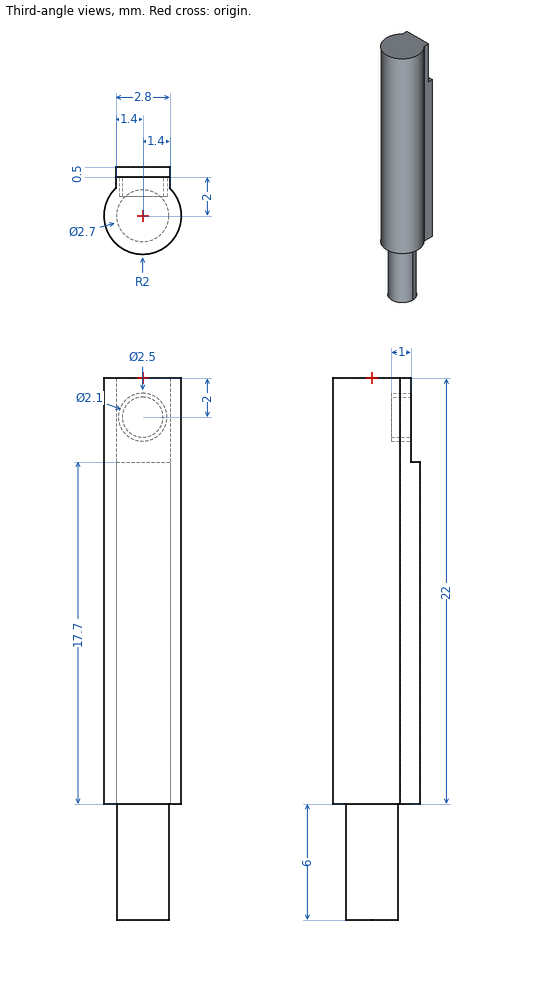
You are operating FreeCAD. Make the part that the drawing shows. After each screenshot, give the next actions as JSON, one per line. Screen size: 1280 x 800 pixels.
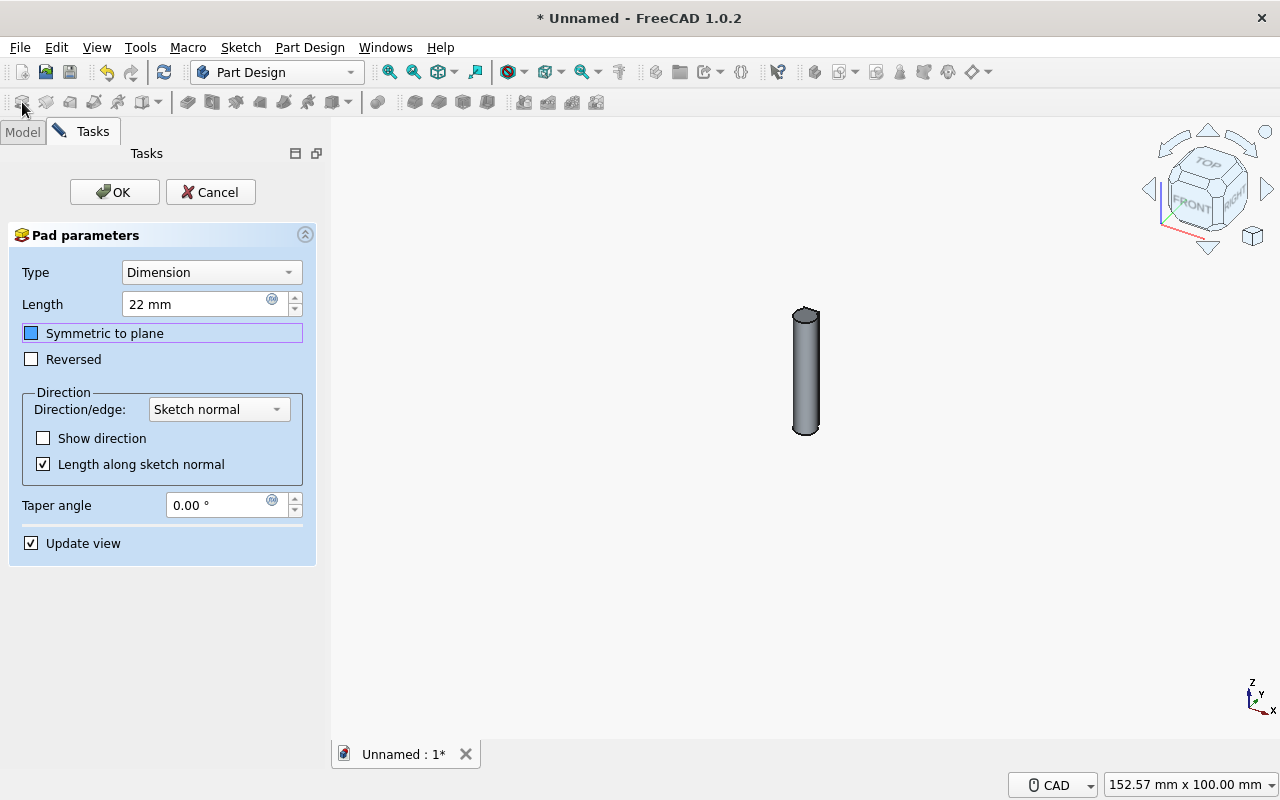
{"action": "left_click", "coordinate": [30, 359]}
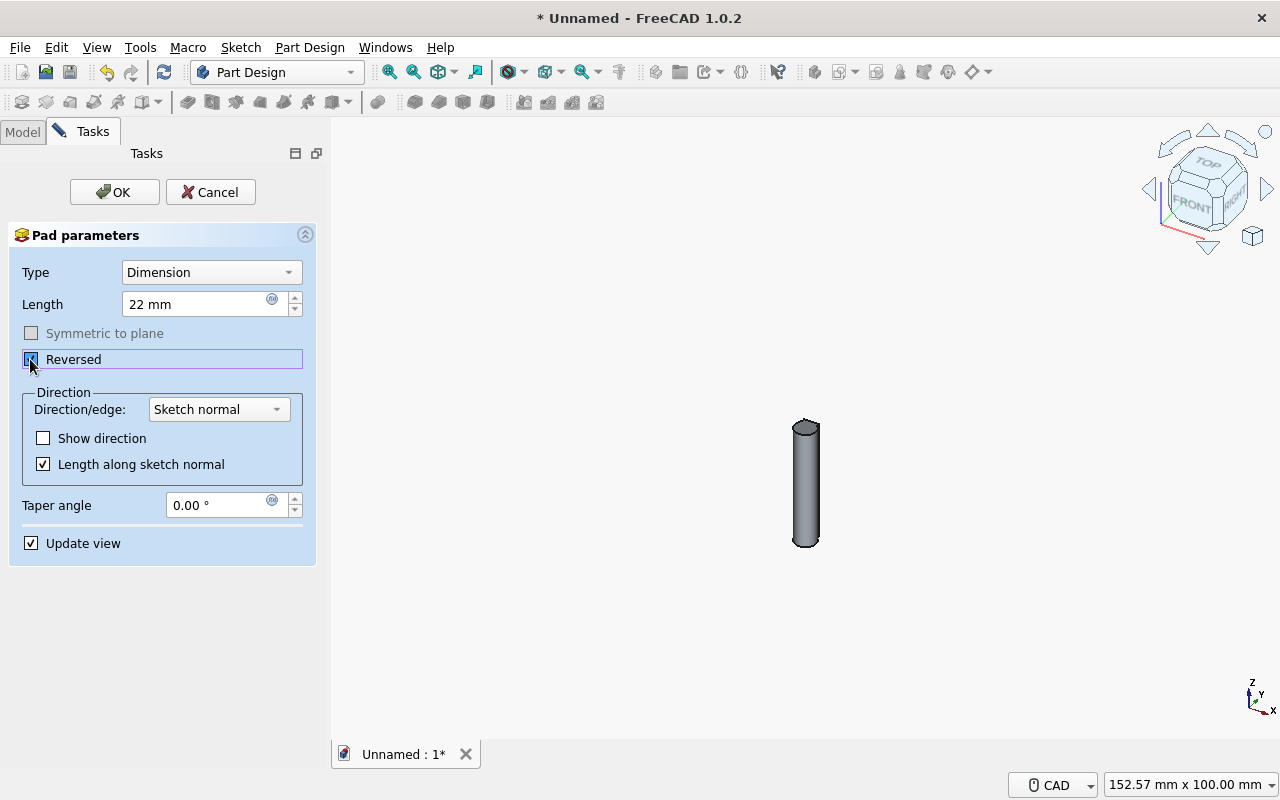
{"action": "left_click", "coordinate": [115, 192]}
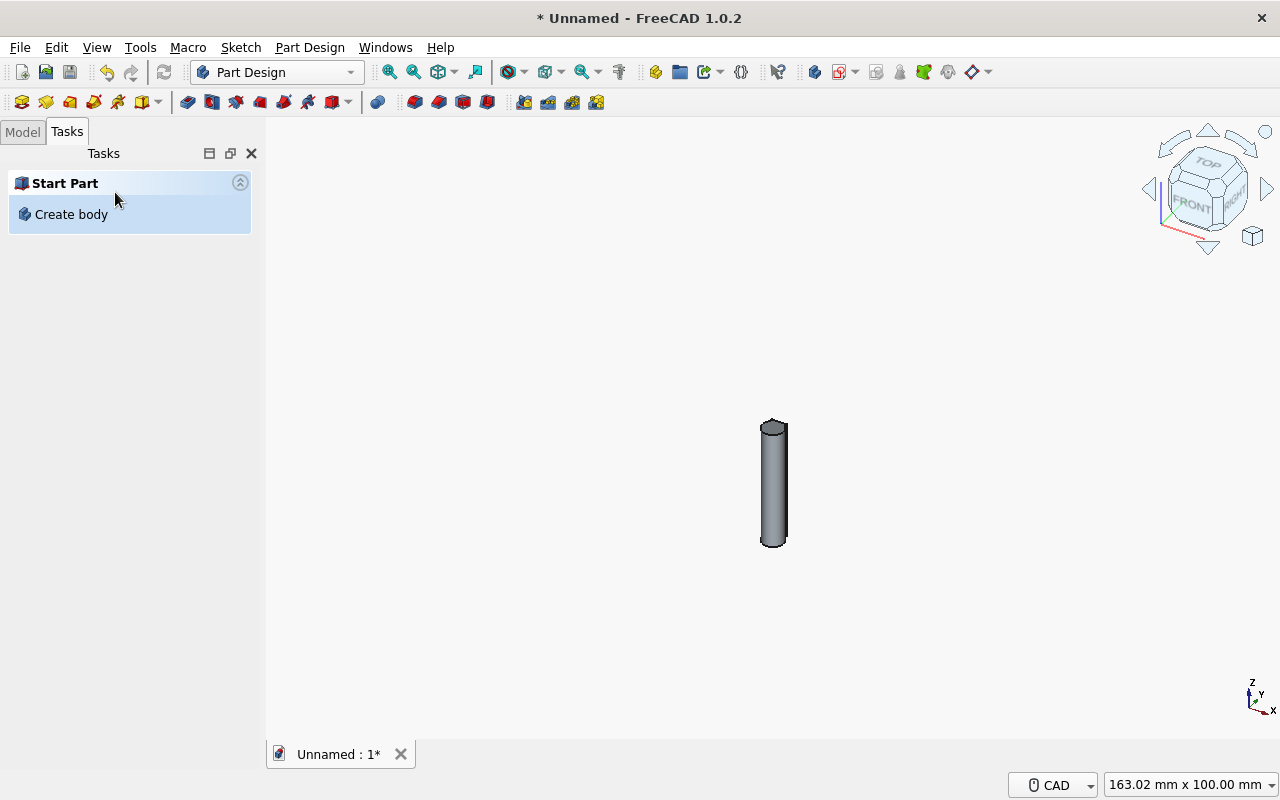
{"action": "left_click", "coordinate": [390, 72]}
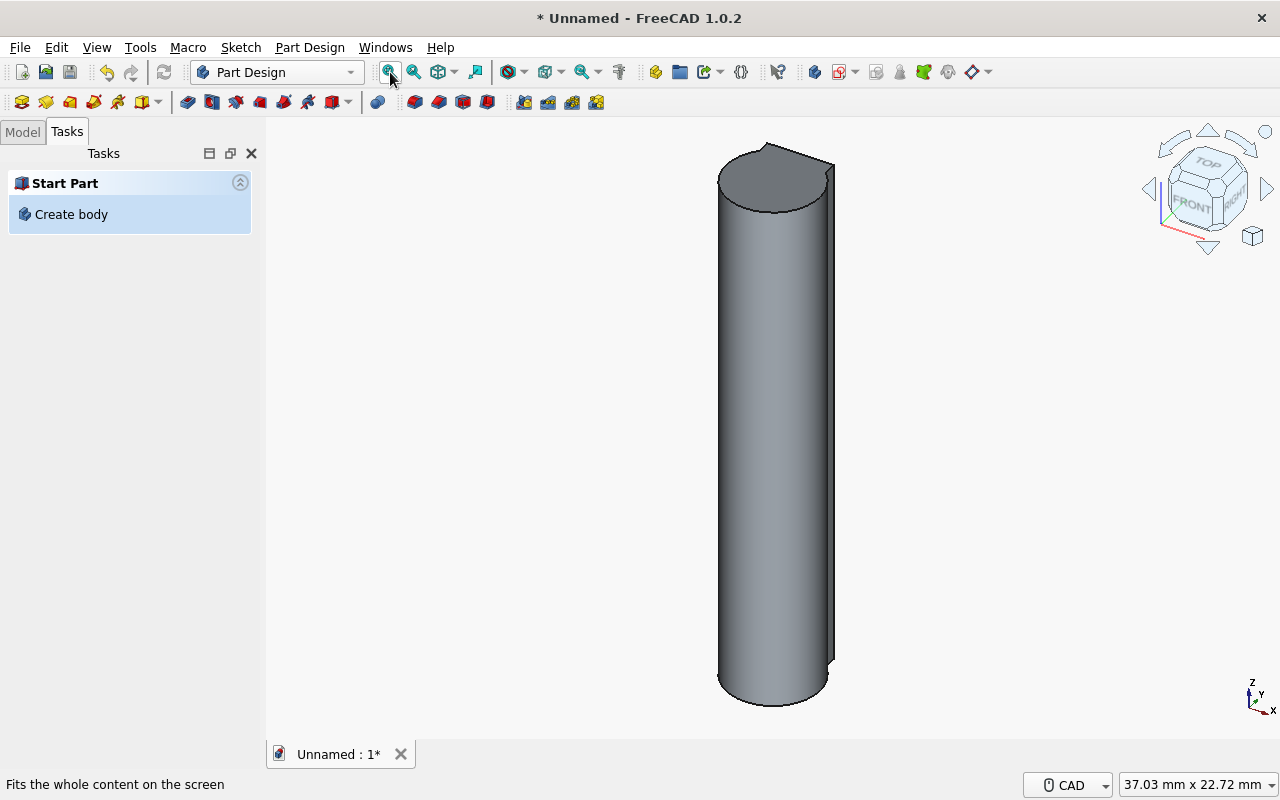
{"action": "key", "text": "5"}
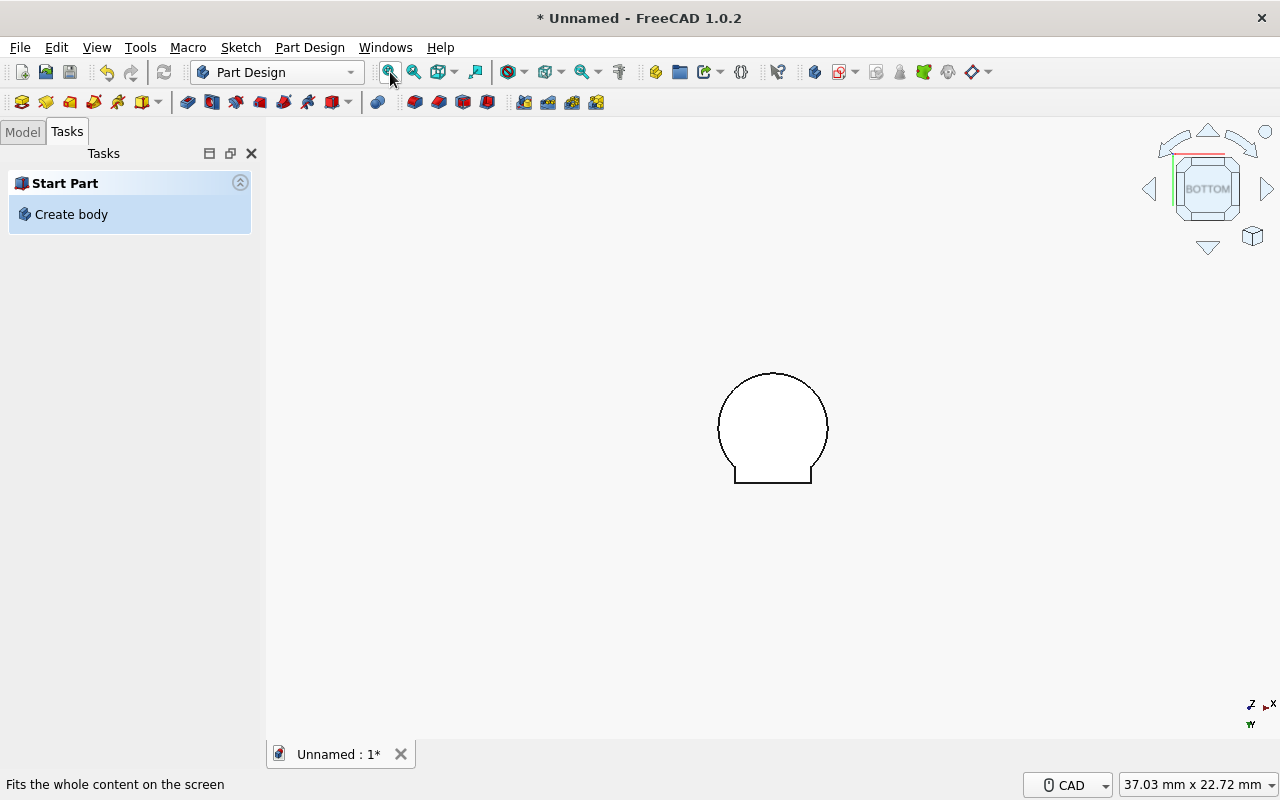
{"action": "left_click", "coordinate": [390, 72]}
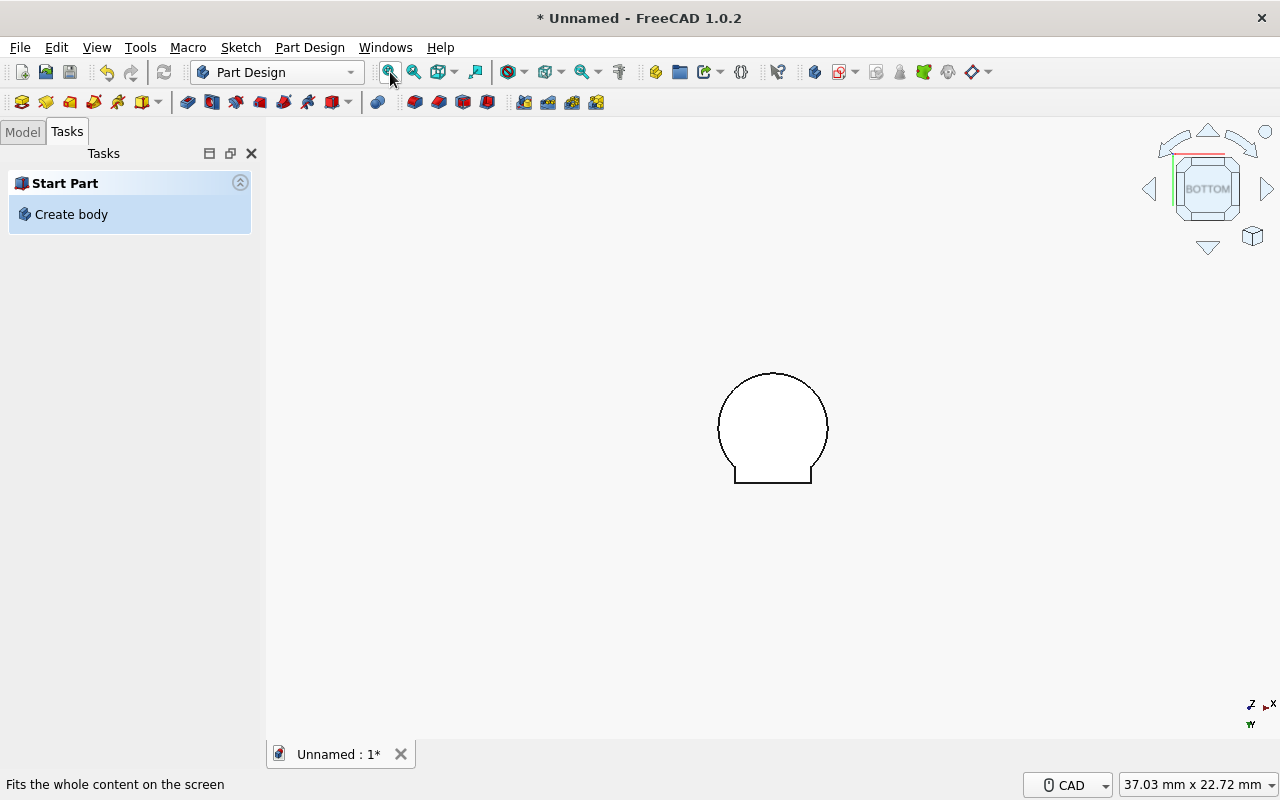
{"action": "left_click", "coordinate": [773, 427]}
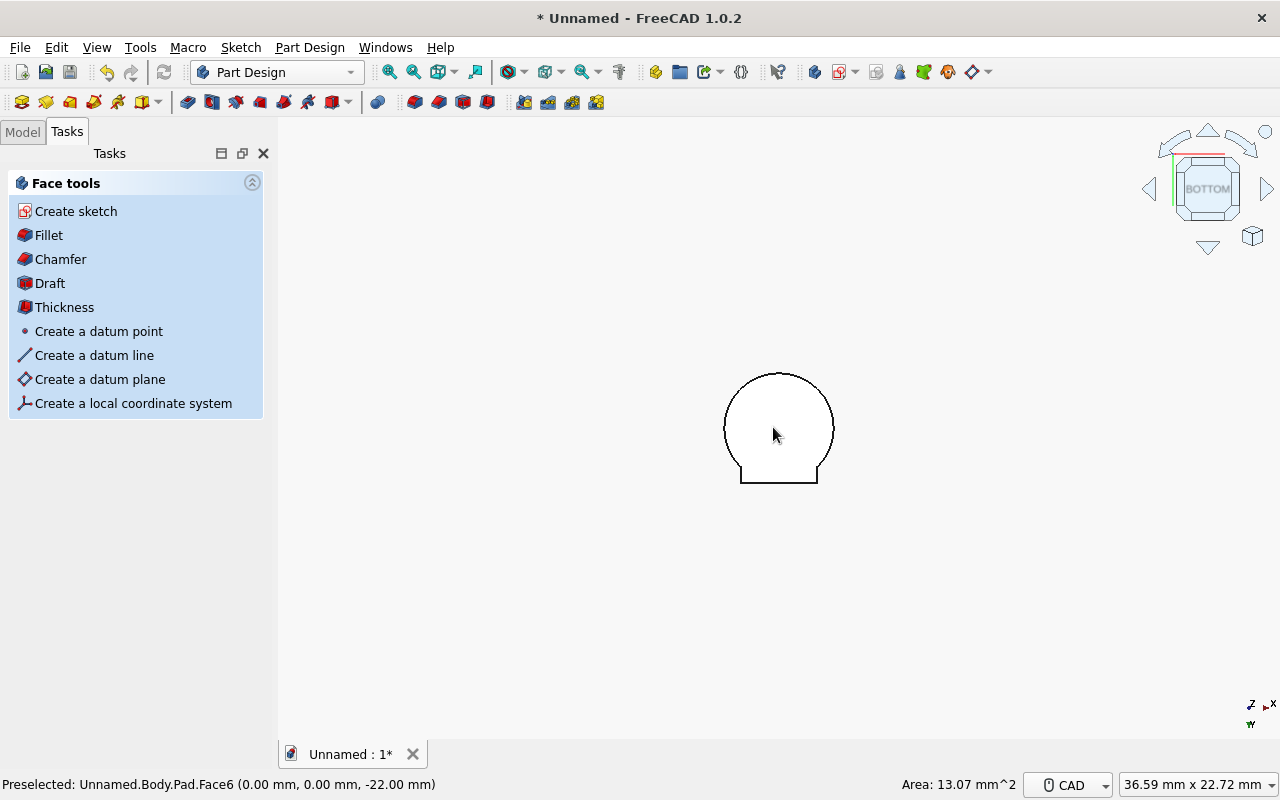
{"action": "left_click", "coordinate": [840, 72]}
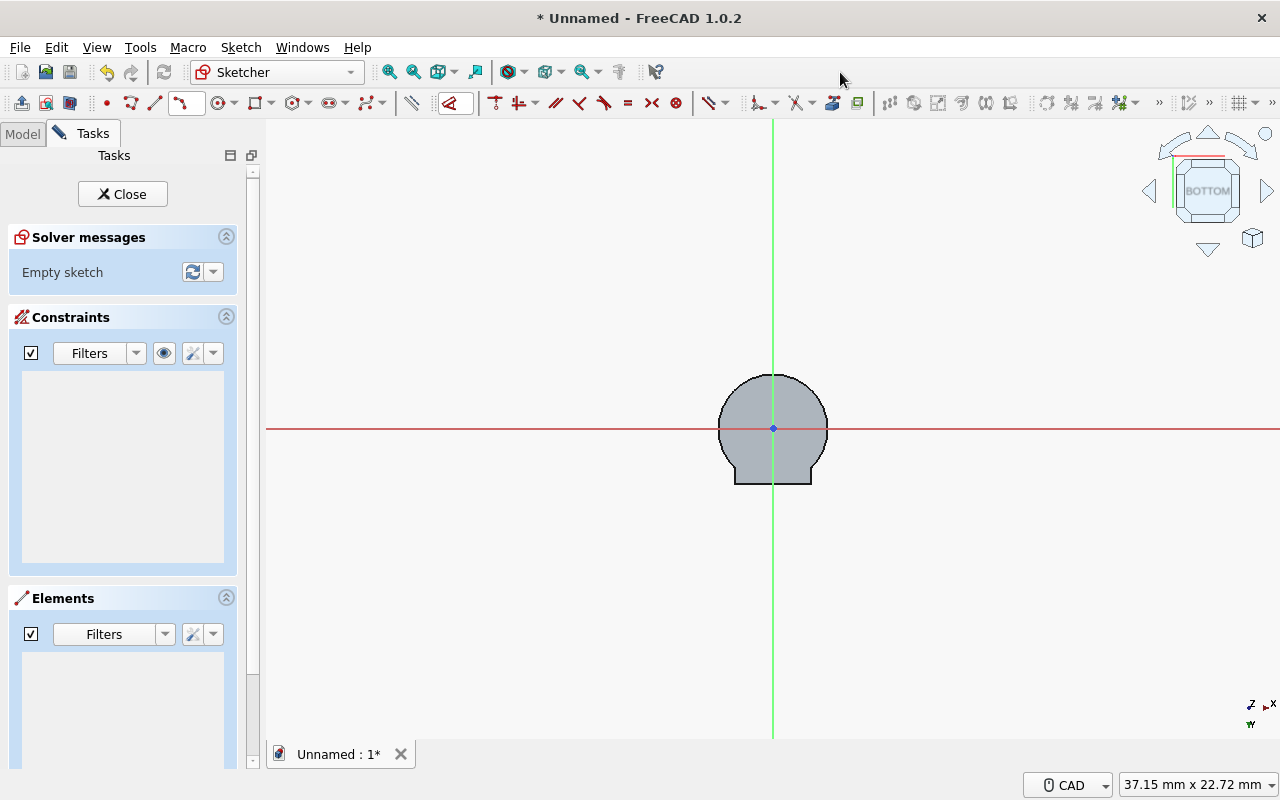
{"action": "scroll", "coordinate": [787, 470], "scroll_direction": "up", "scroll_amount": 9}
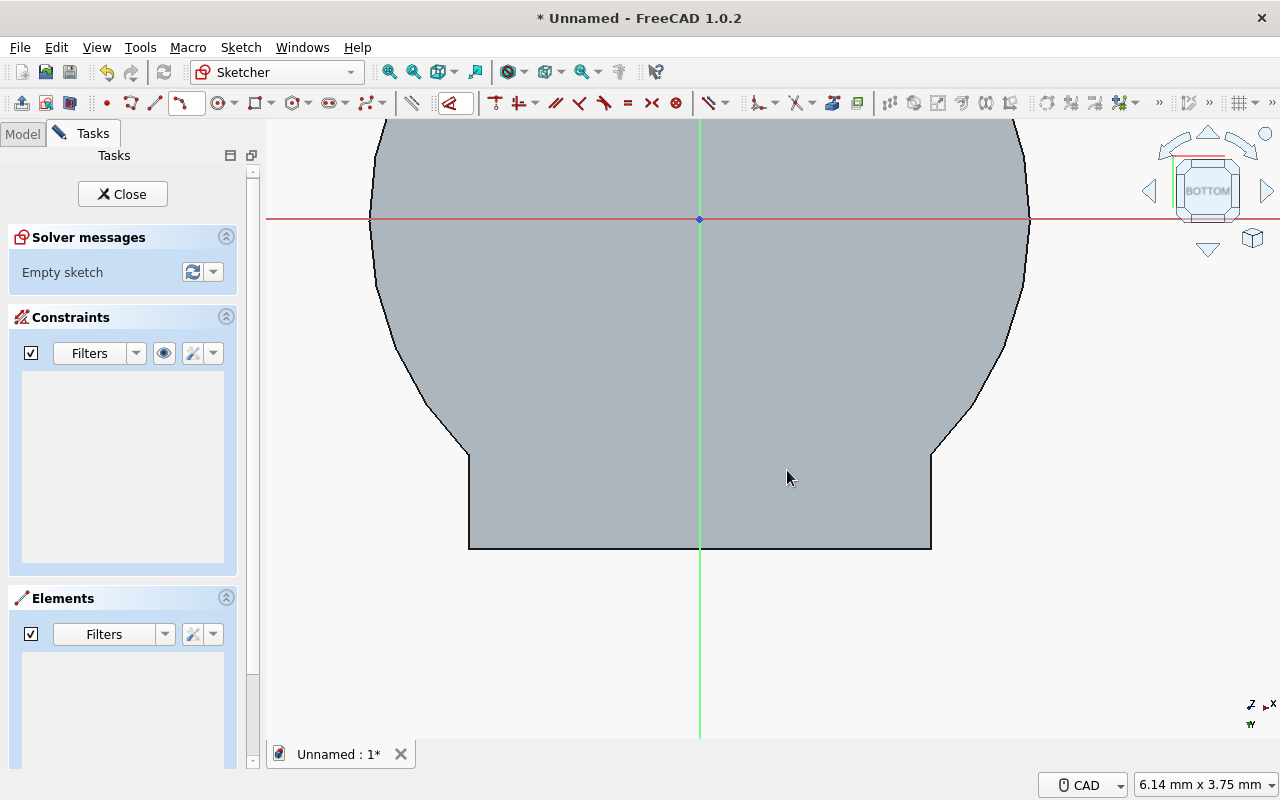
{"action": "key", "text": "g r"}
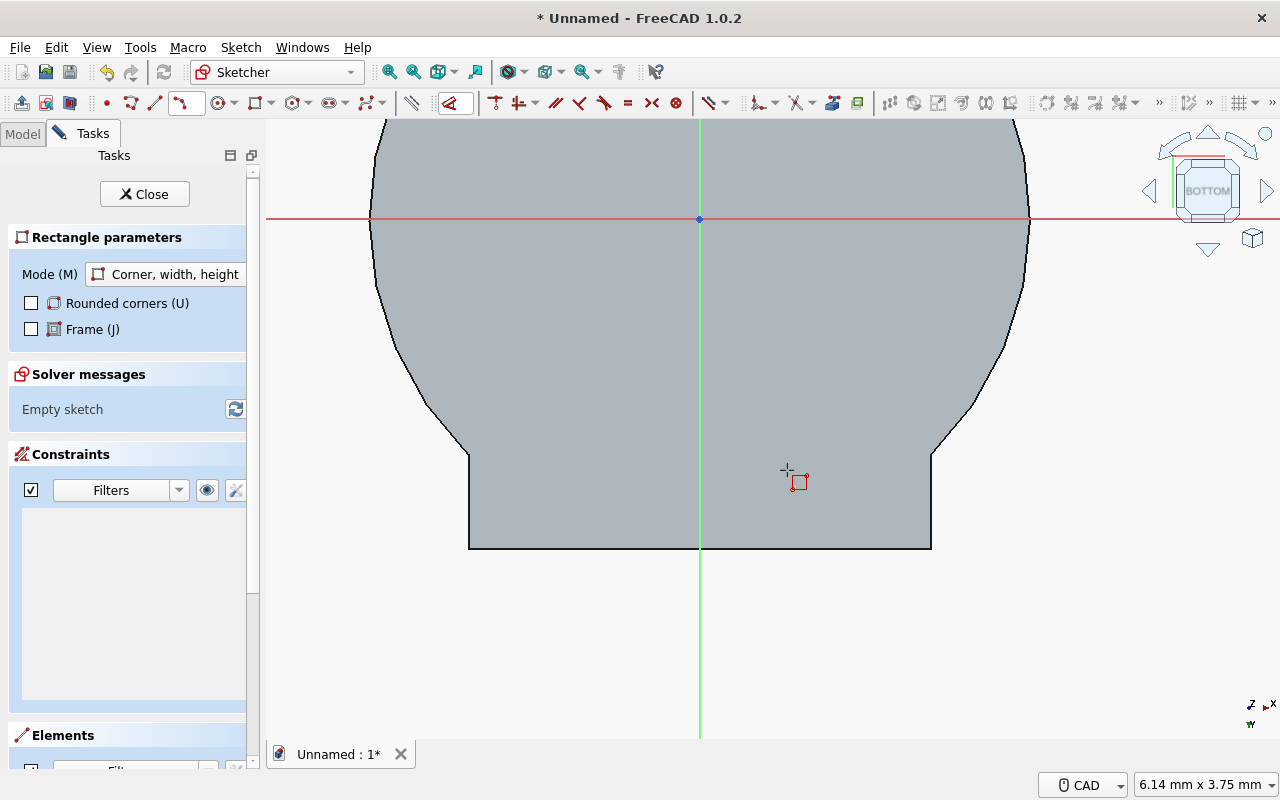
{"action": "left_click", "coordinate": [469, 549]}
{"action": "left_click", "coordinate": [931, 632]}
{"action": "key", "text": "Escape"}